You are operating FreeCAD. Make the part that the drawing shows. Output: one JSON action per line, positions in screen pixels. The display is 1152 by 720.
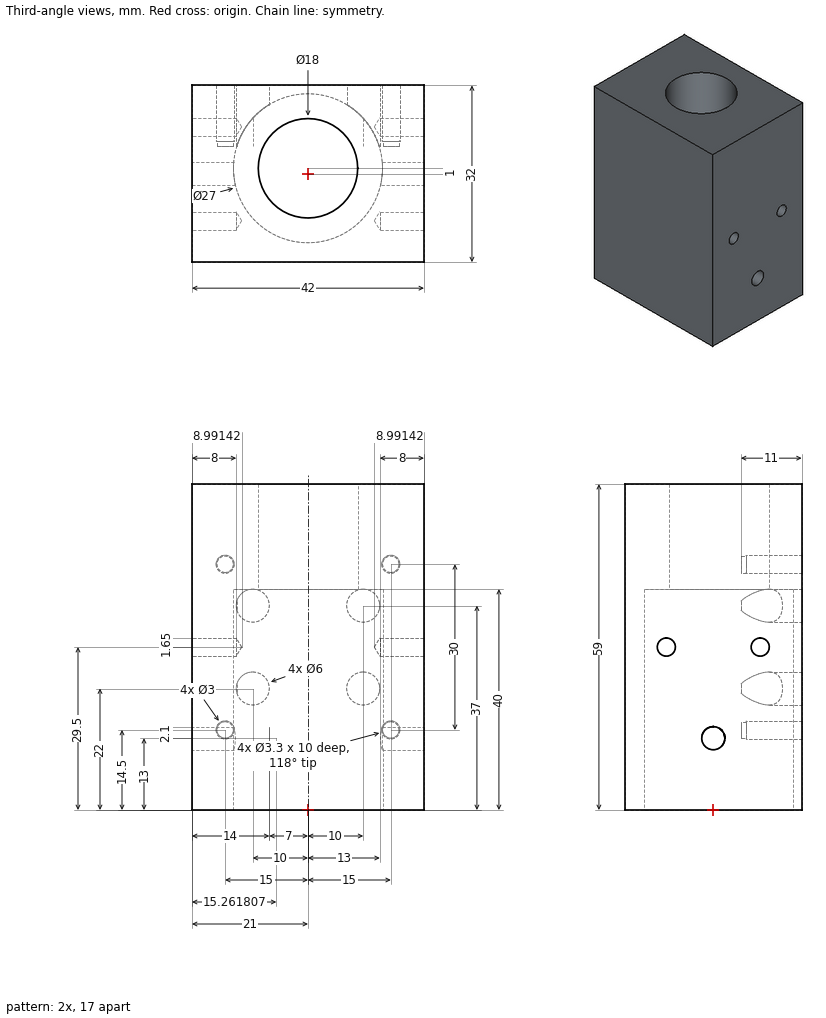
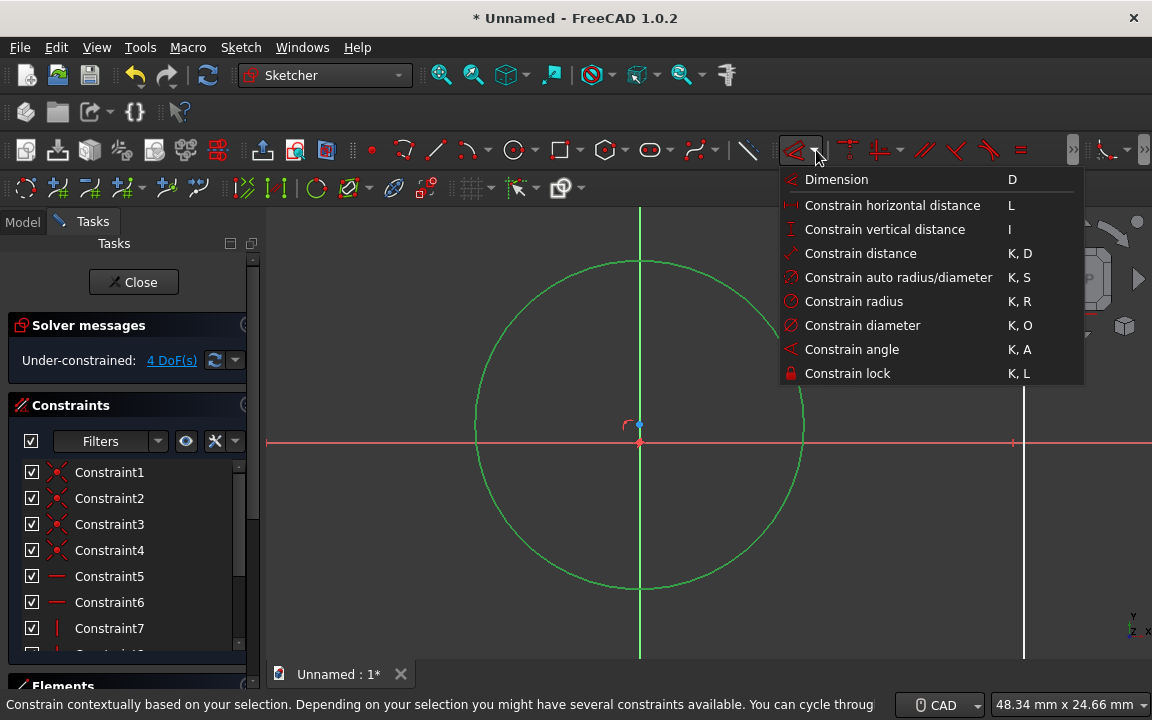
{"action": "left_click", "coordinate": [932, 325]}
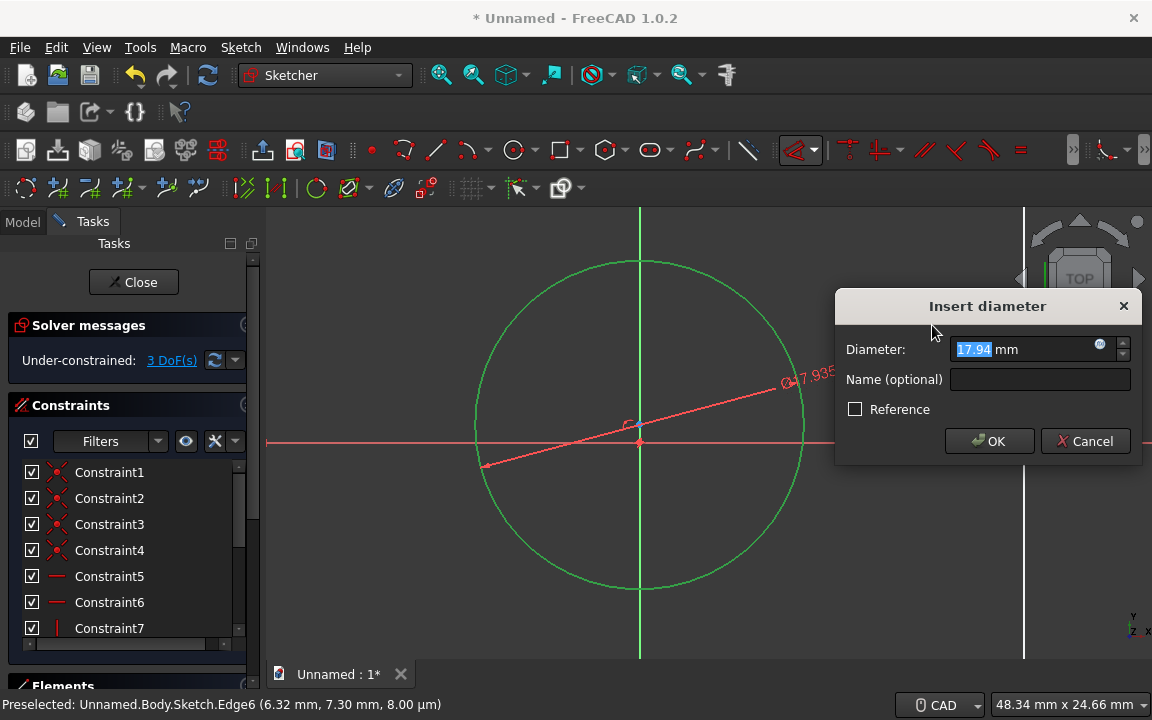
{"action": "type", "text": "18"}
{"action": "key", "text": "Return"}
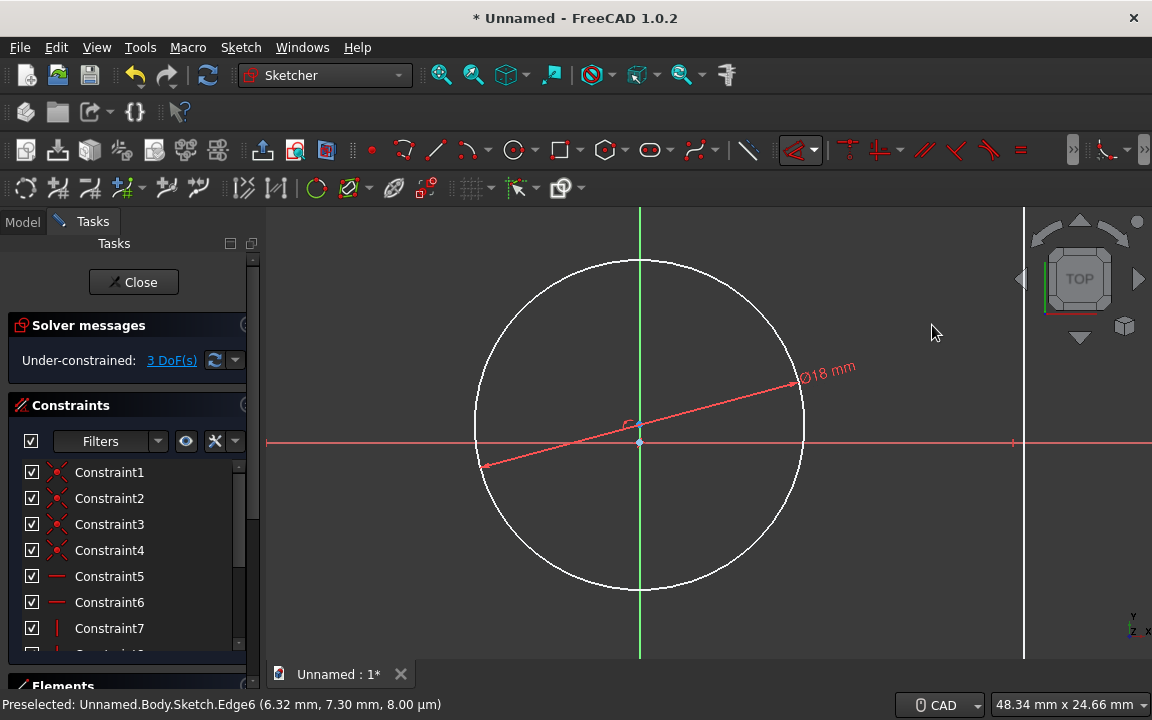
{"action": "scroll", "coordinate": [640, 425], "scroll_direction": "up", "scroll_amount": 4}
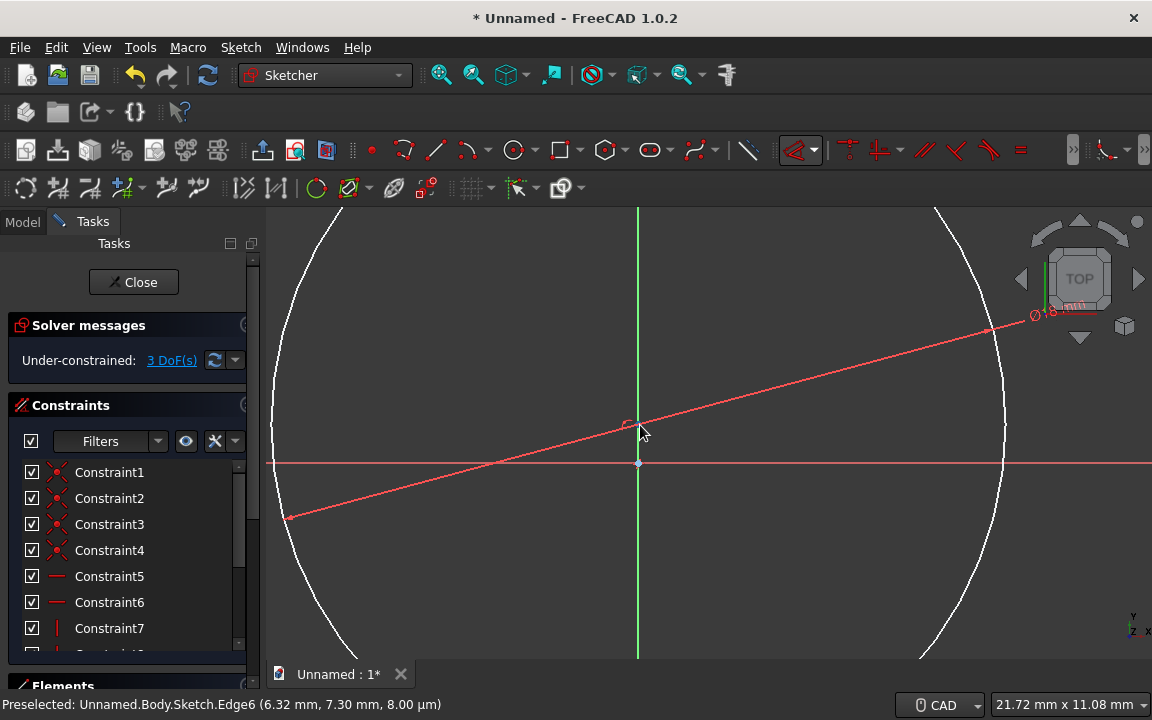
{"action": "left_click", "coordinate": [638, 424]}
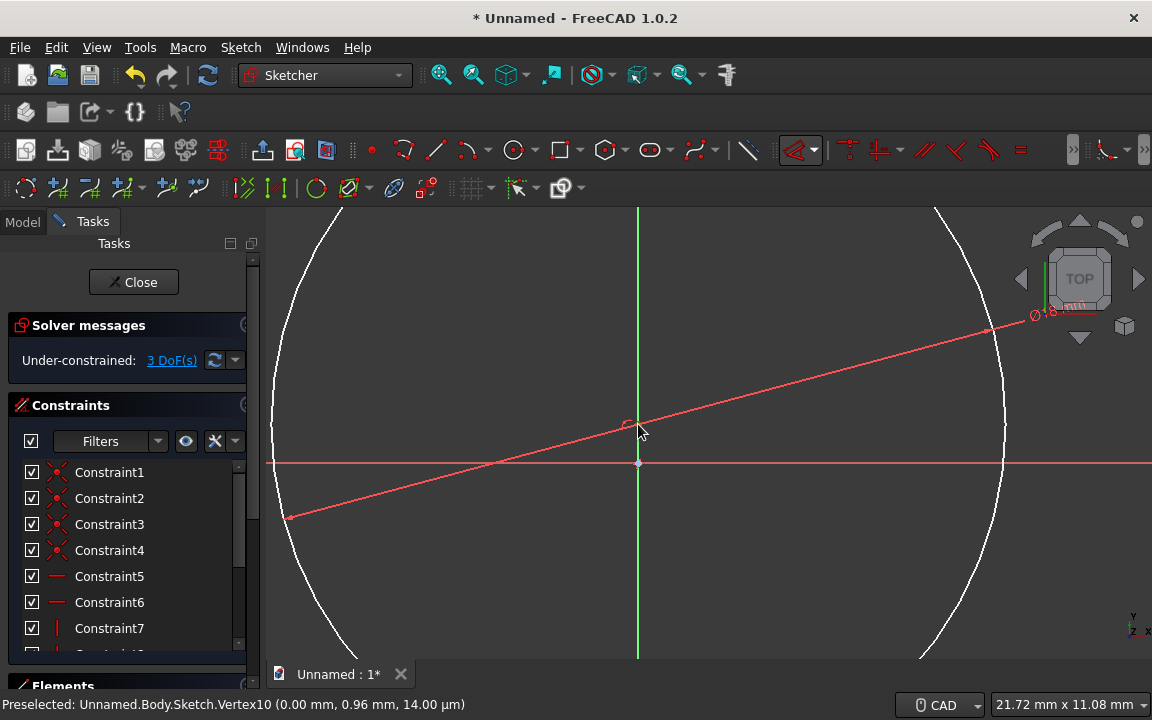
{"action": "left_click", "coordinate": [816, 150]}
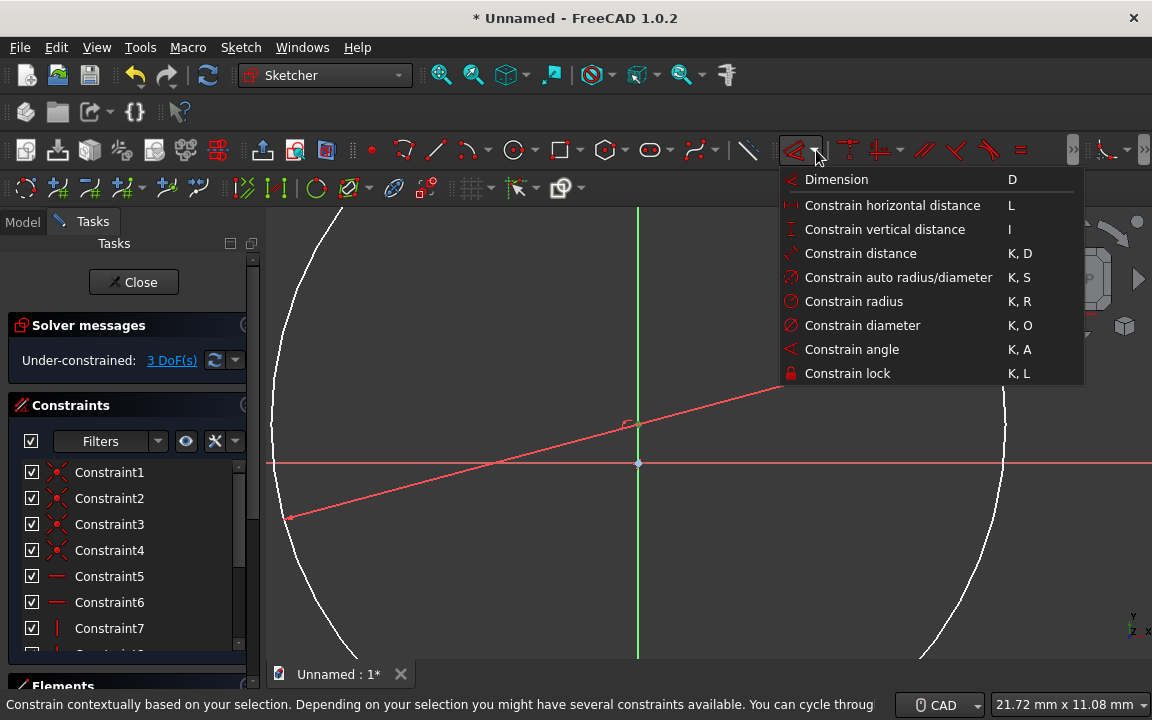
{"action": "left_click", "coordinate": [932, 229]}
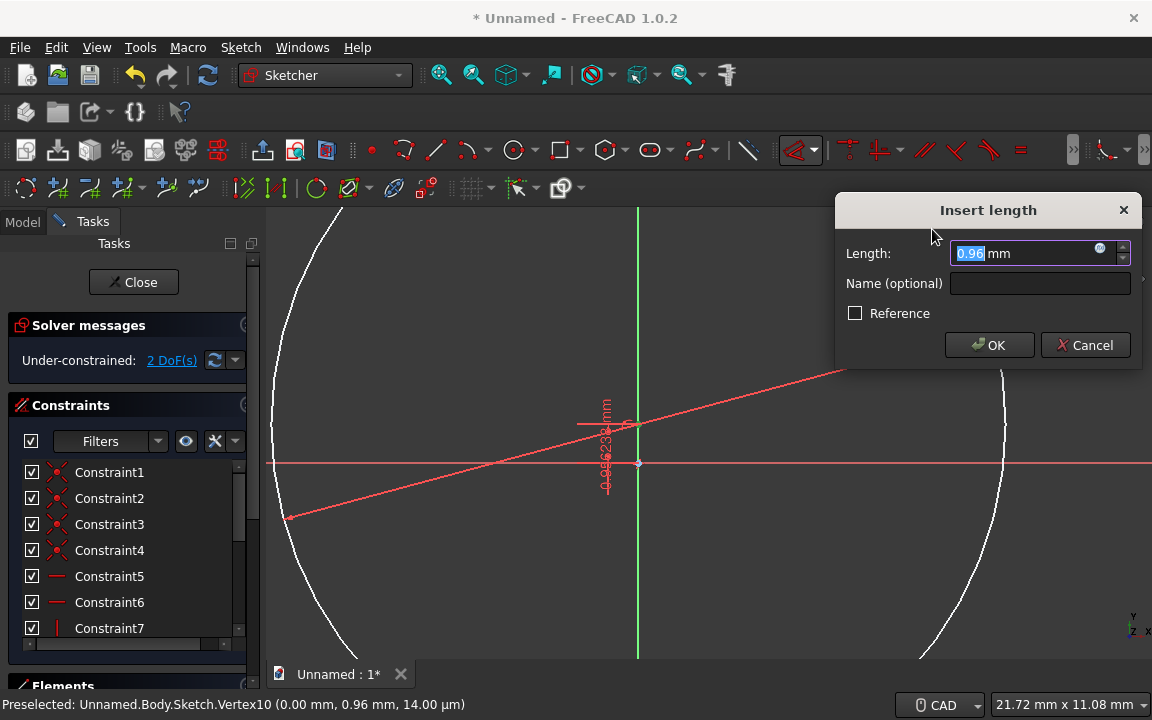
{"action": "type", "text": "1"}
{"action": "key", "text": "Return"}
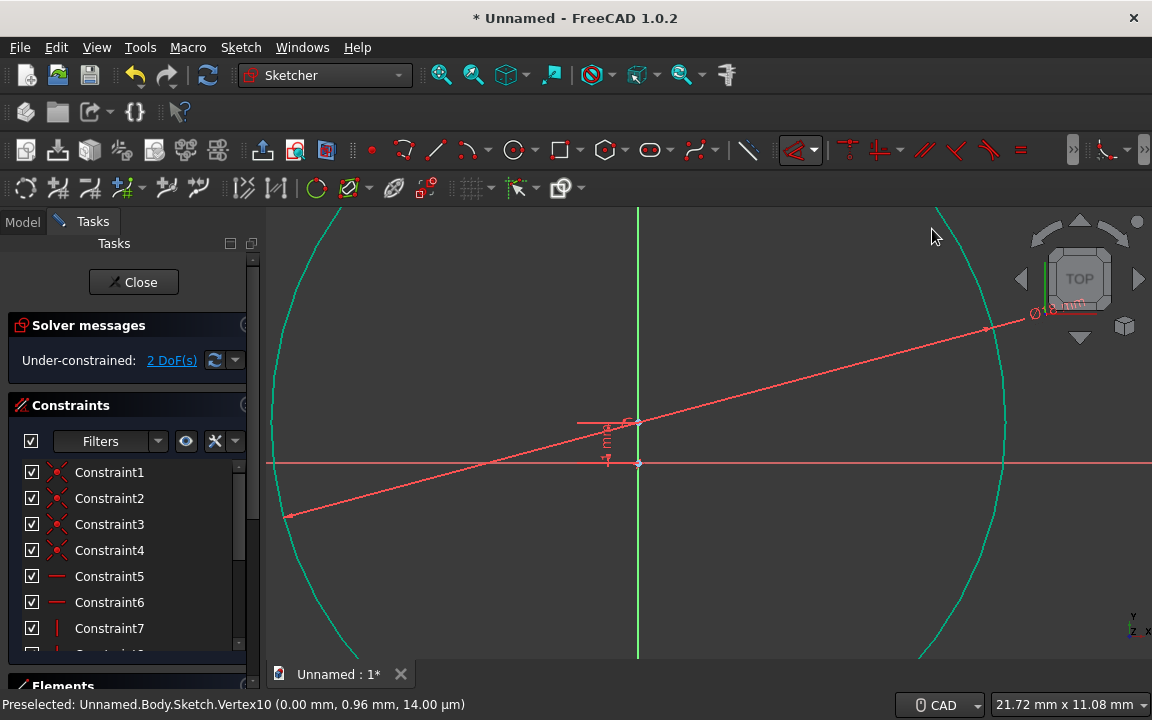
{"action": "scroll", "coordinate": [641, 425], "scroll_direction": "down", "scroll_amount": 8}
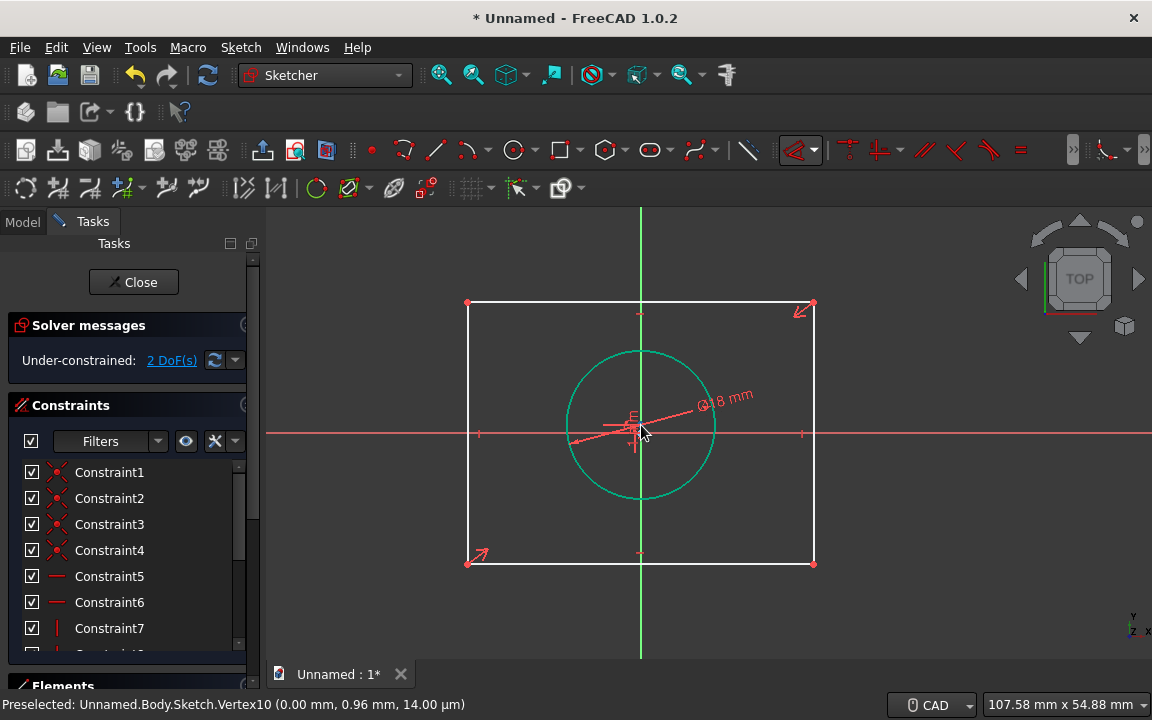
{"action": "left_click", "coordinate": [572, 564]}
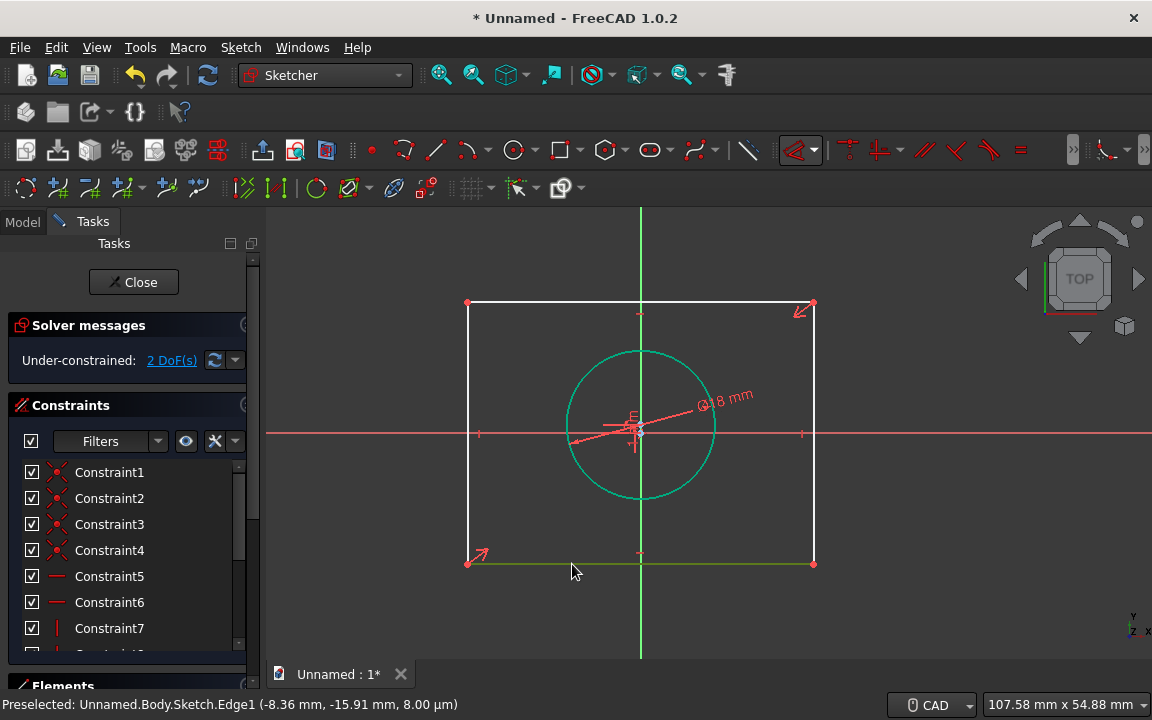
{"action": "left_click", "coordinate": [816, 150]}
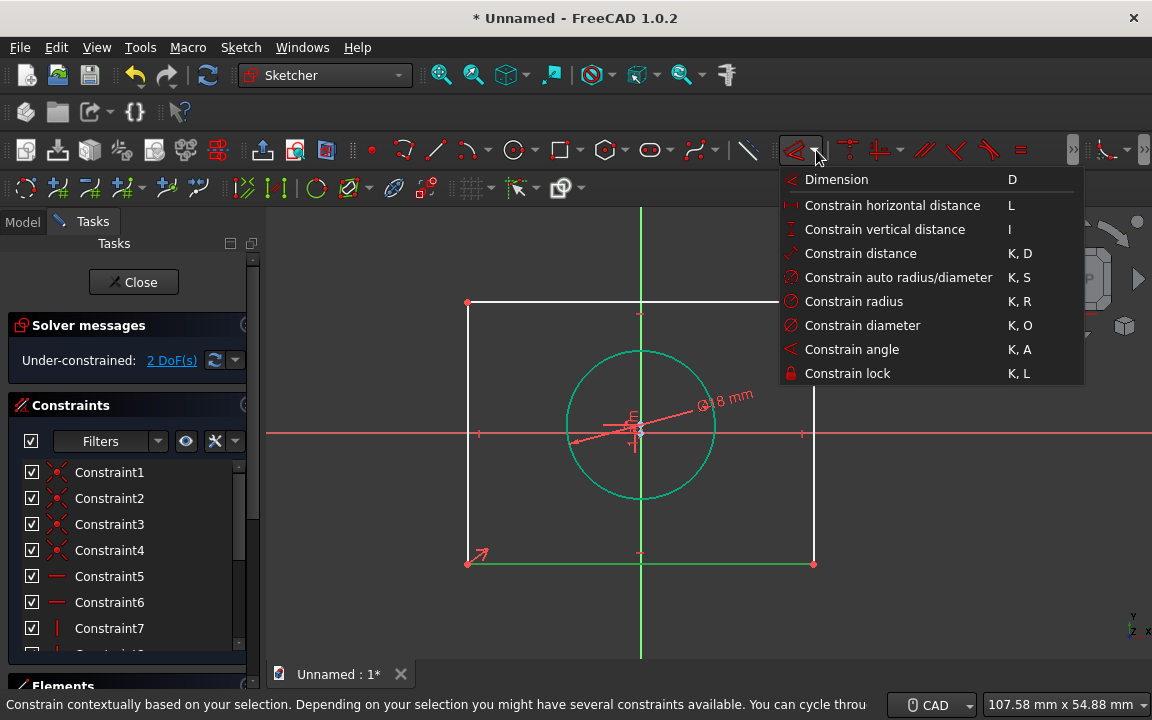
{"action": "left_click", "coordinate": [932, 205]}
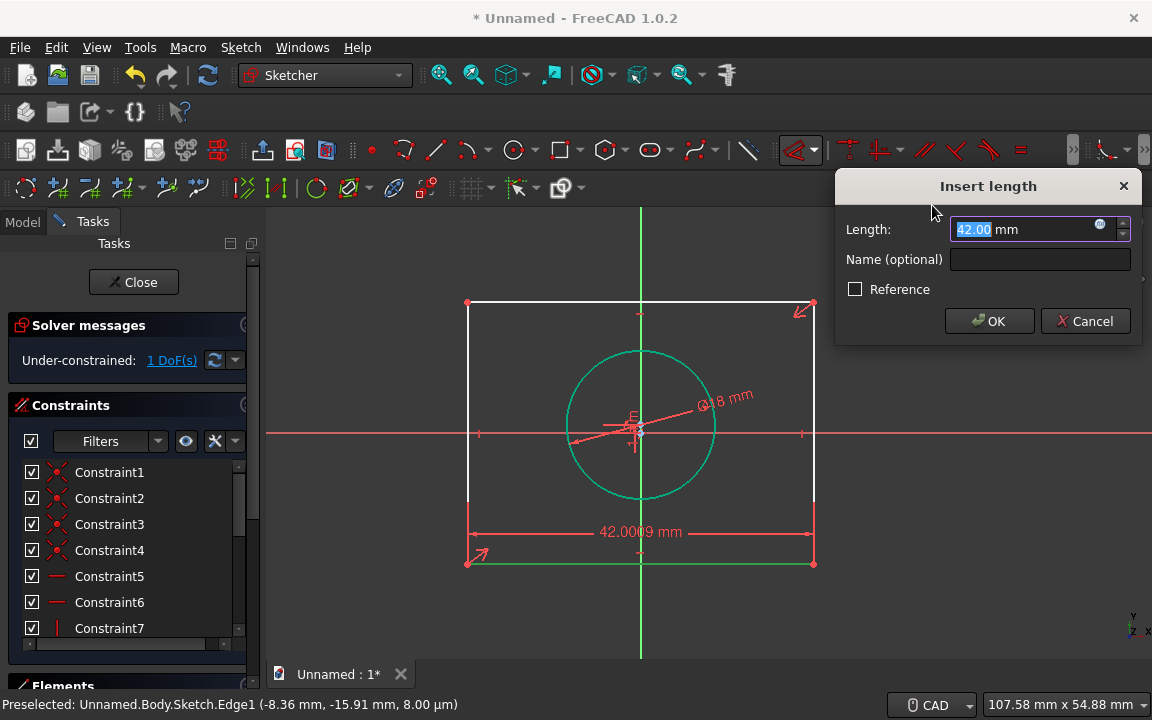
{"action": "type", "text": "42"}
{"action": "key", "text": "Return"}